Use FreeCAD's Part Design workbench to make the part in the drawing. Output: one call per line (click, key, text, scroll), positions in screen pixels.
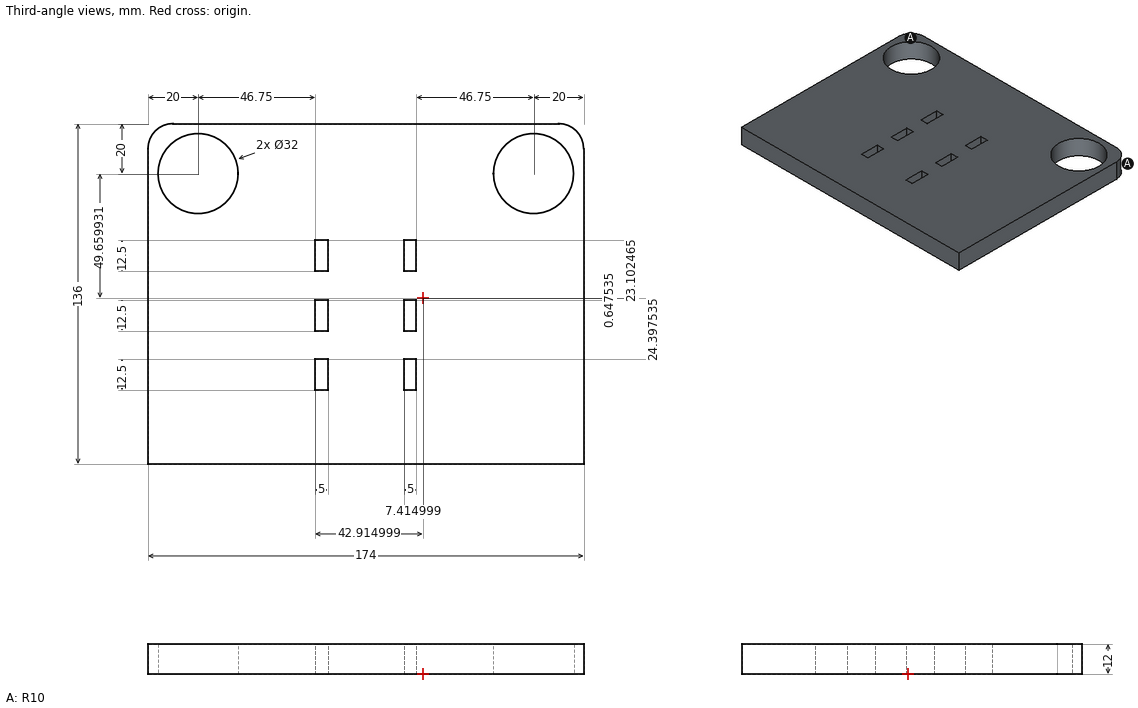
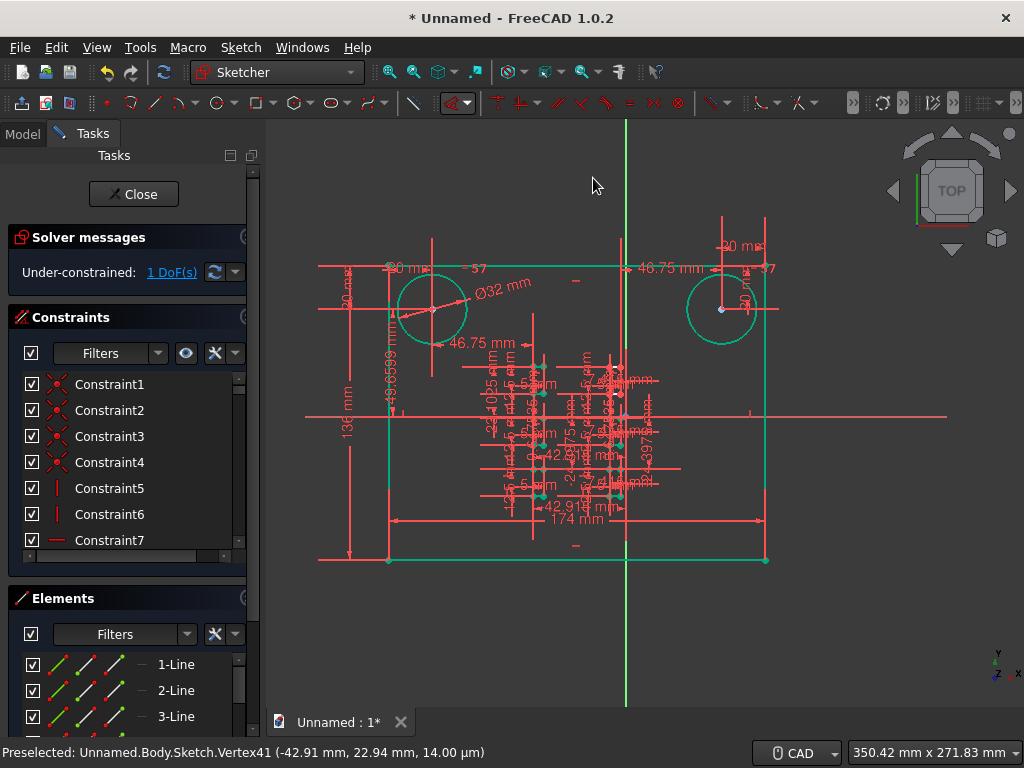
click(610, 367)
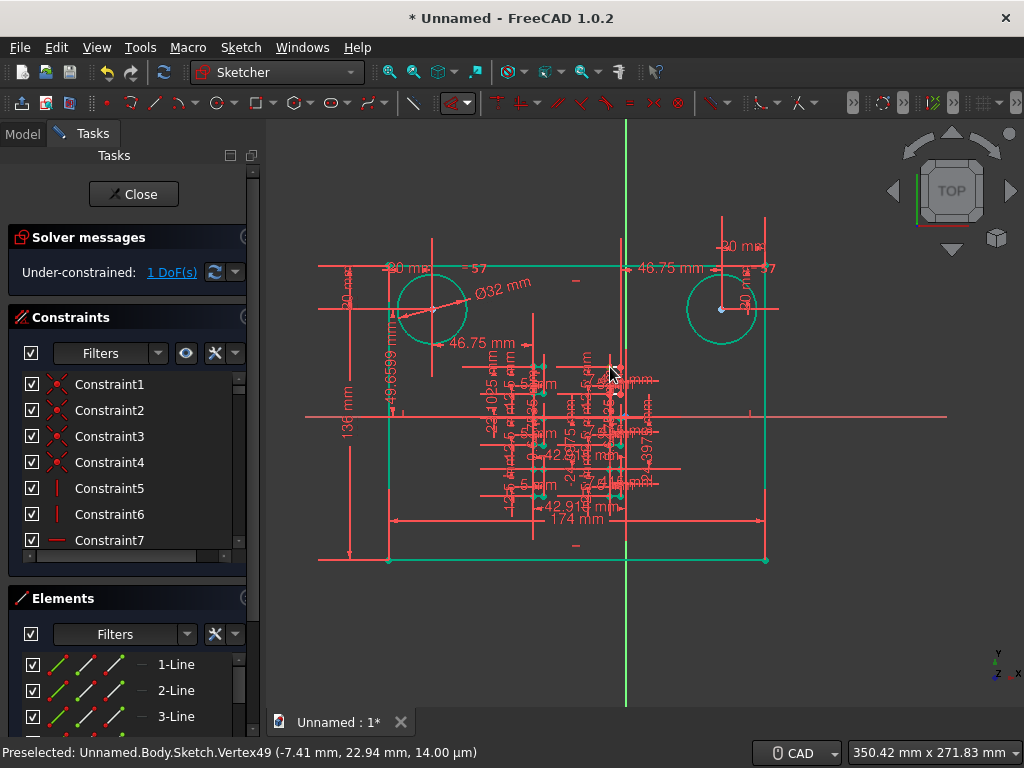
key(i)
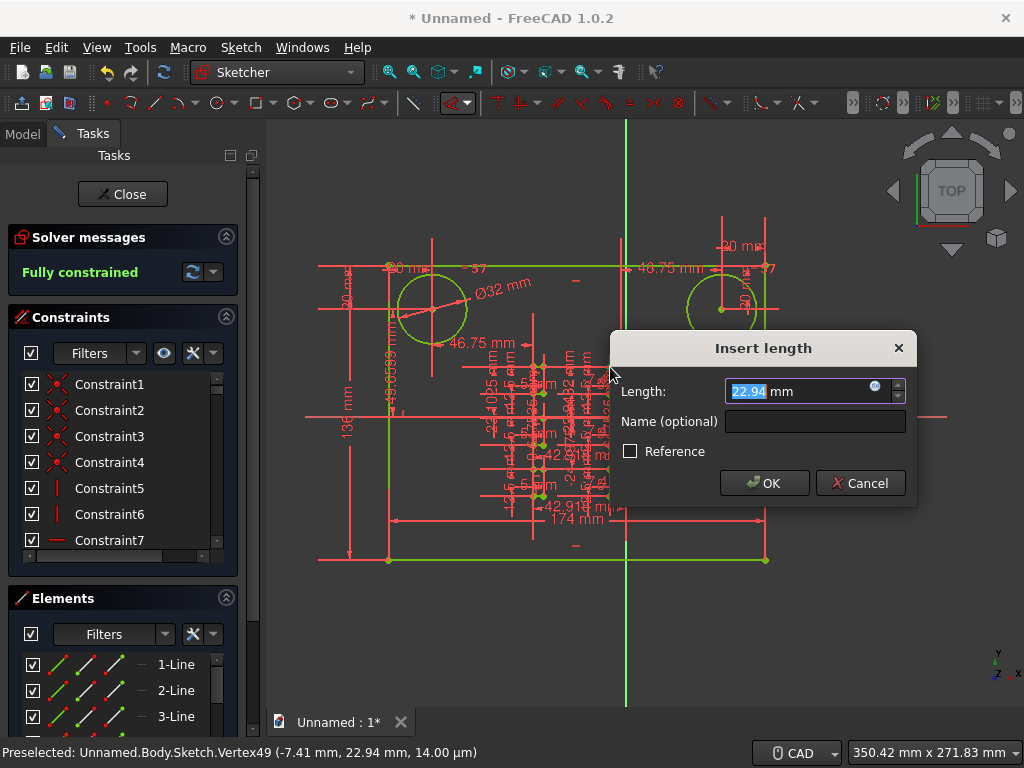
text(23.102465)
key(Return)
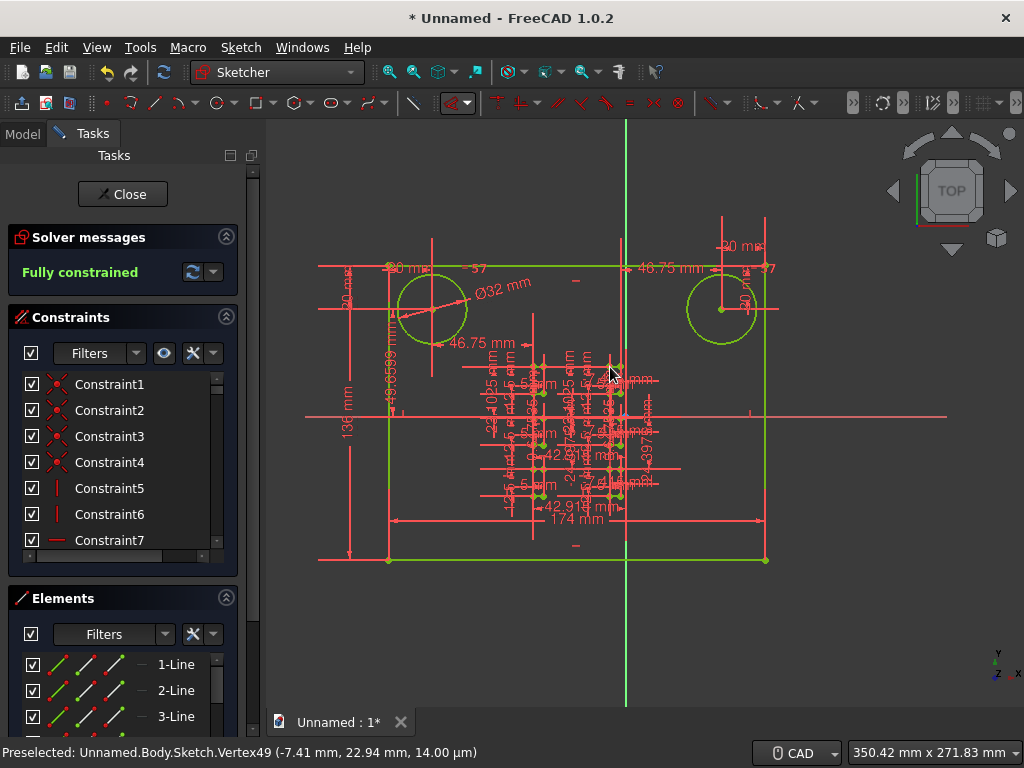
click(123, 194)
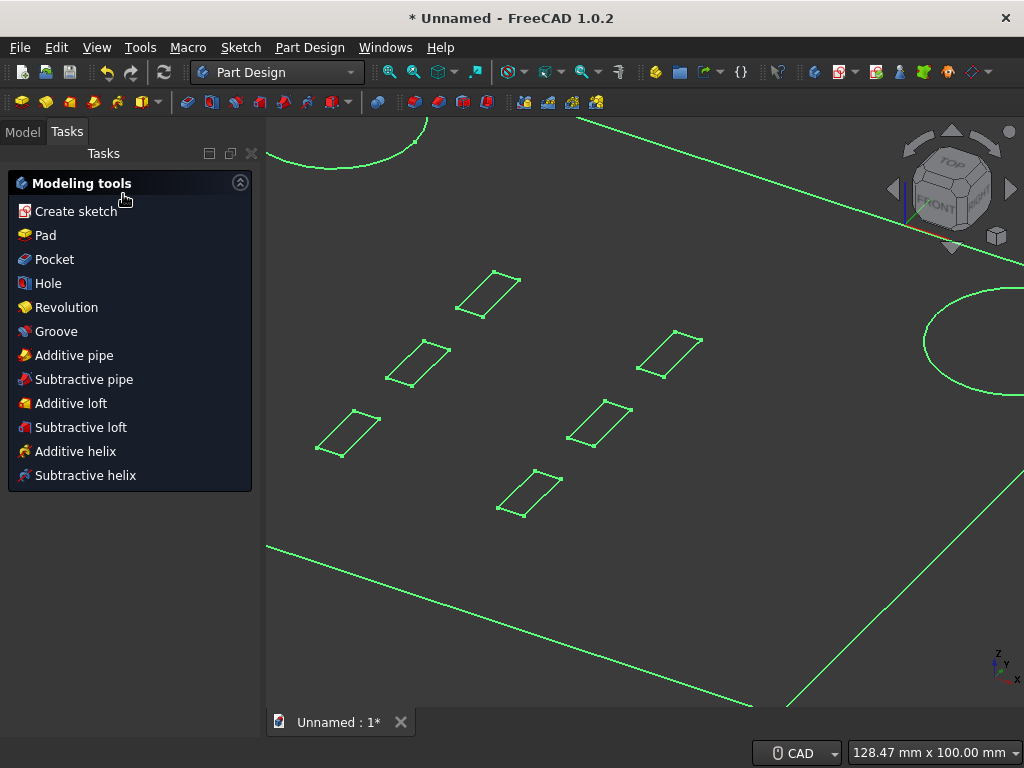
click(22, 102)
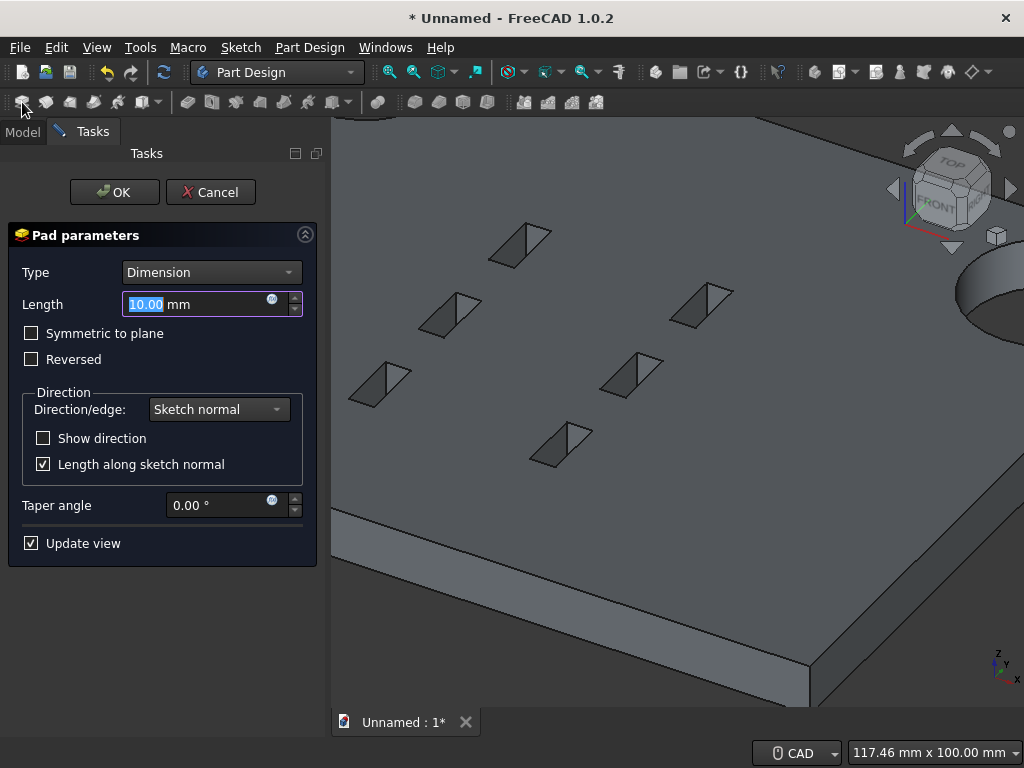
text(12)
key(Tab)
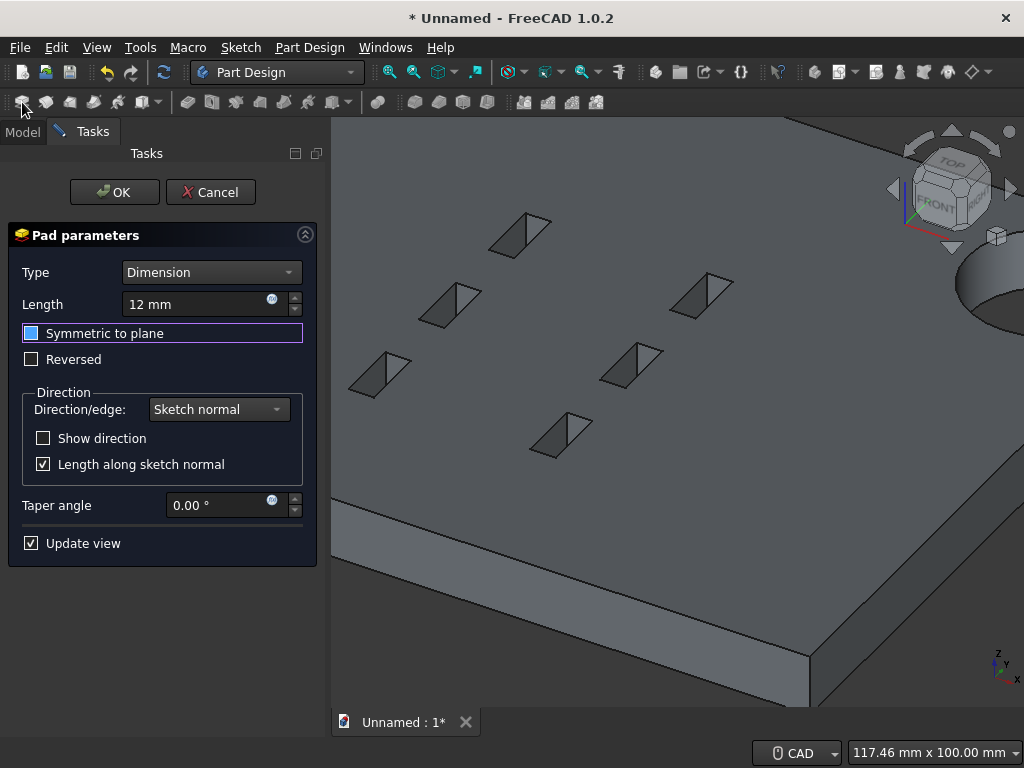
click(115, 192)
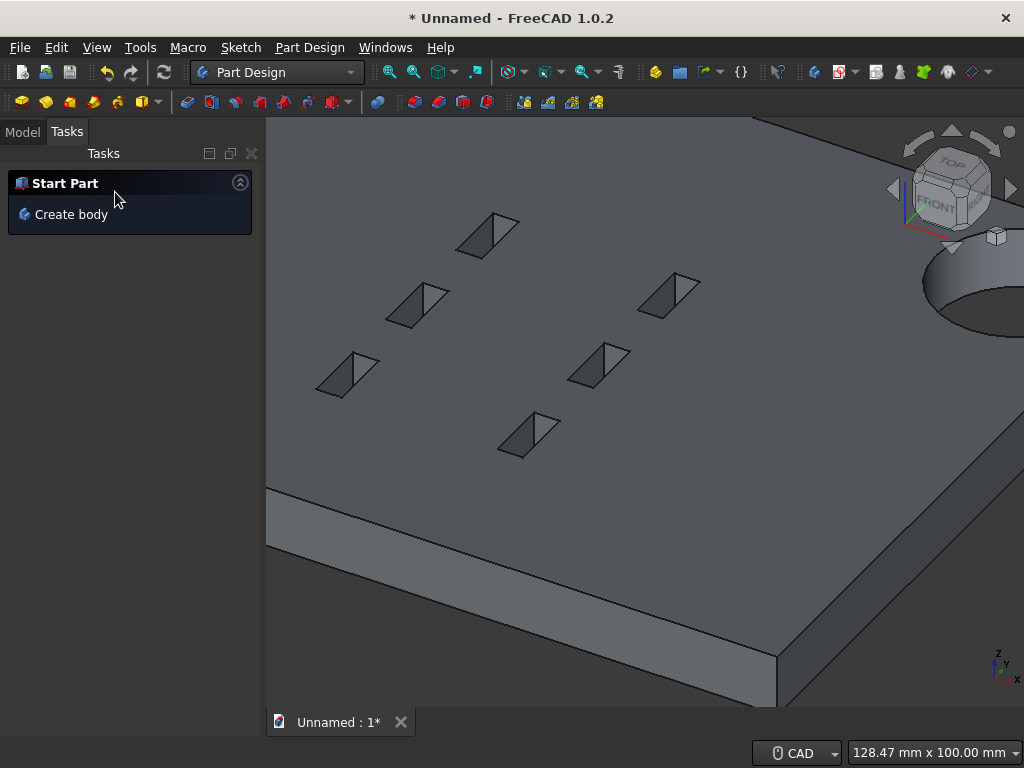
click(390, 72)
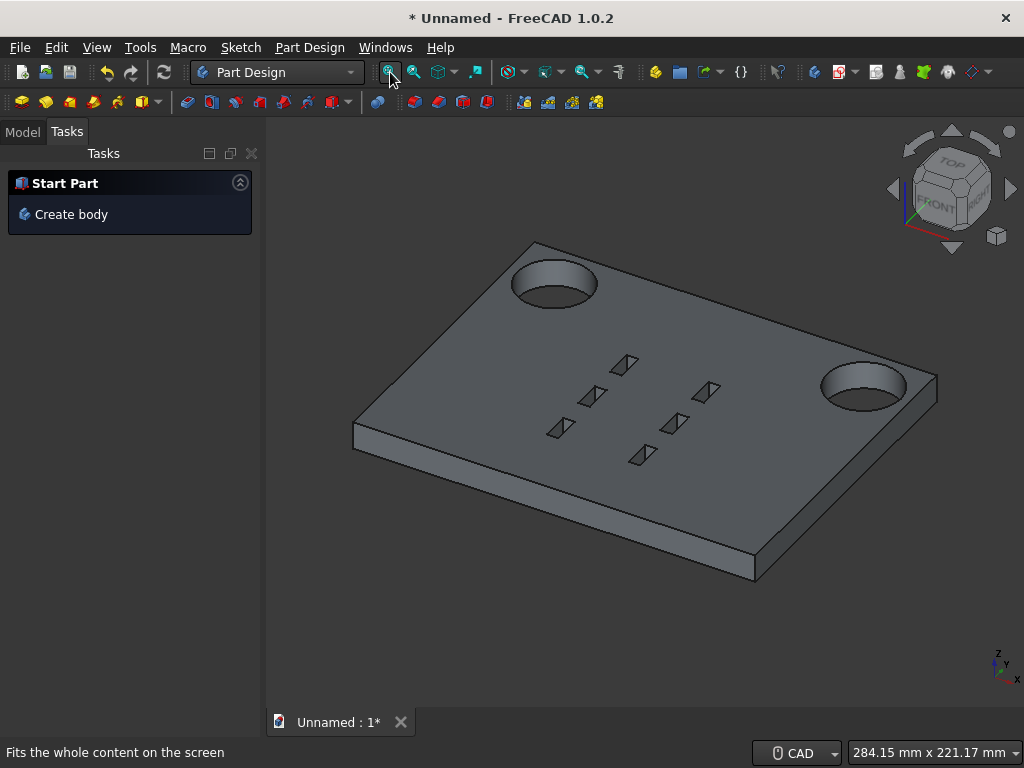
key(0)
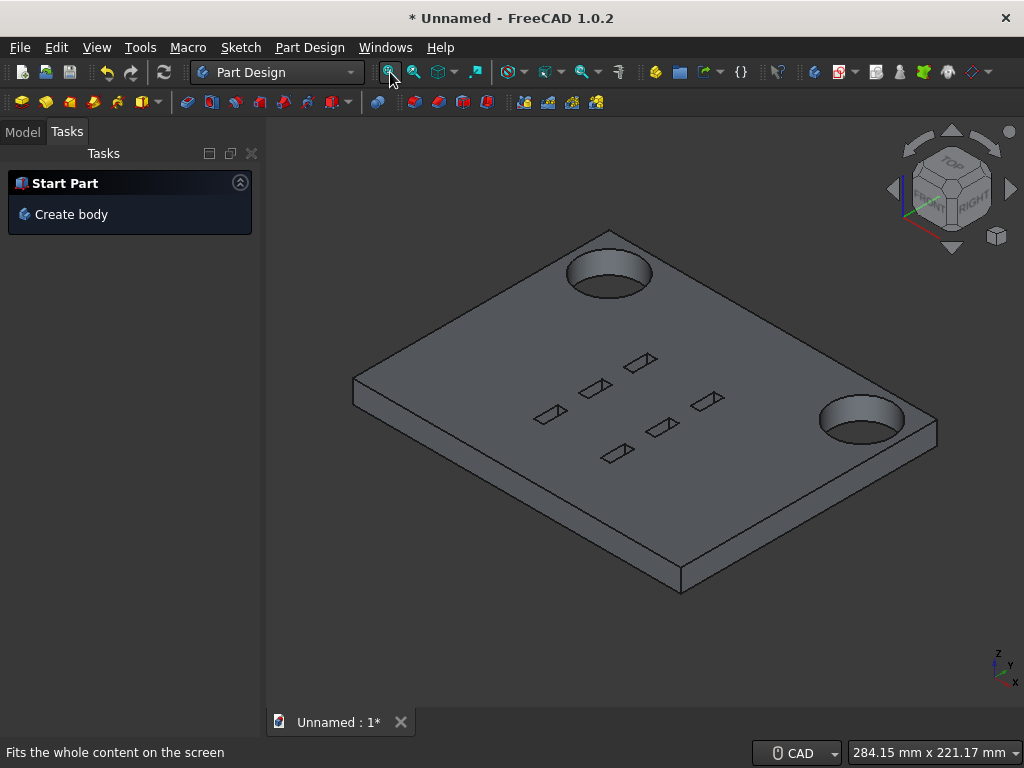
key(2)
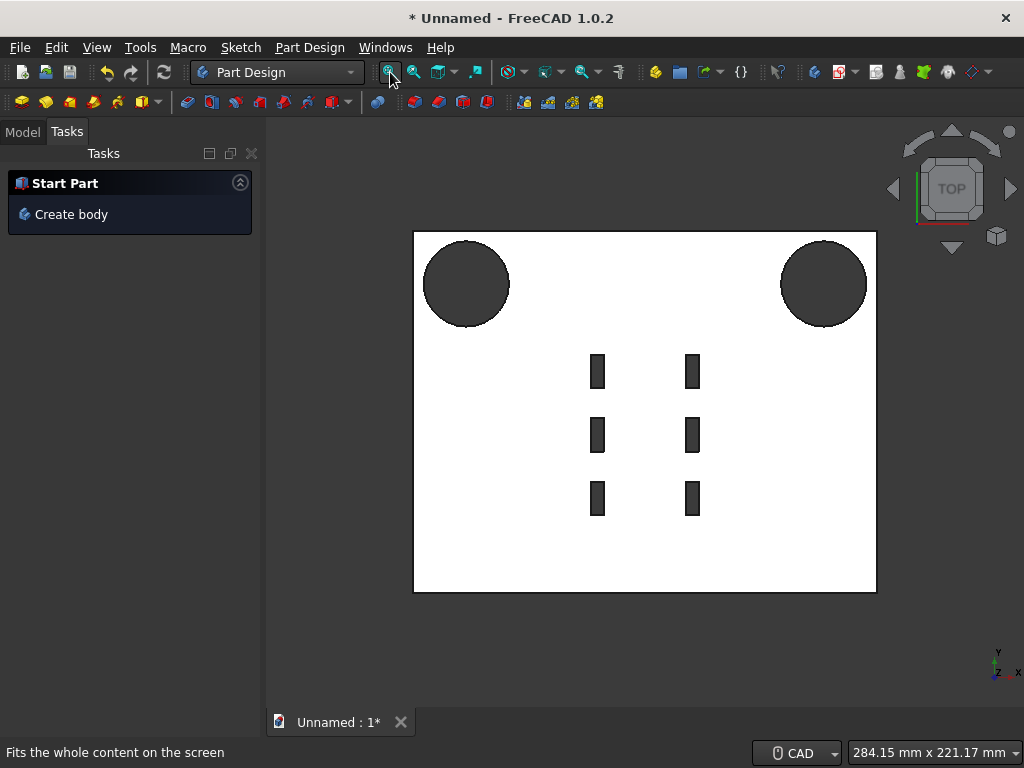
key(1)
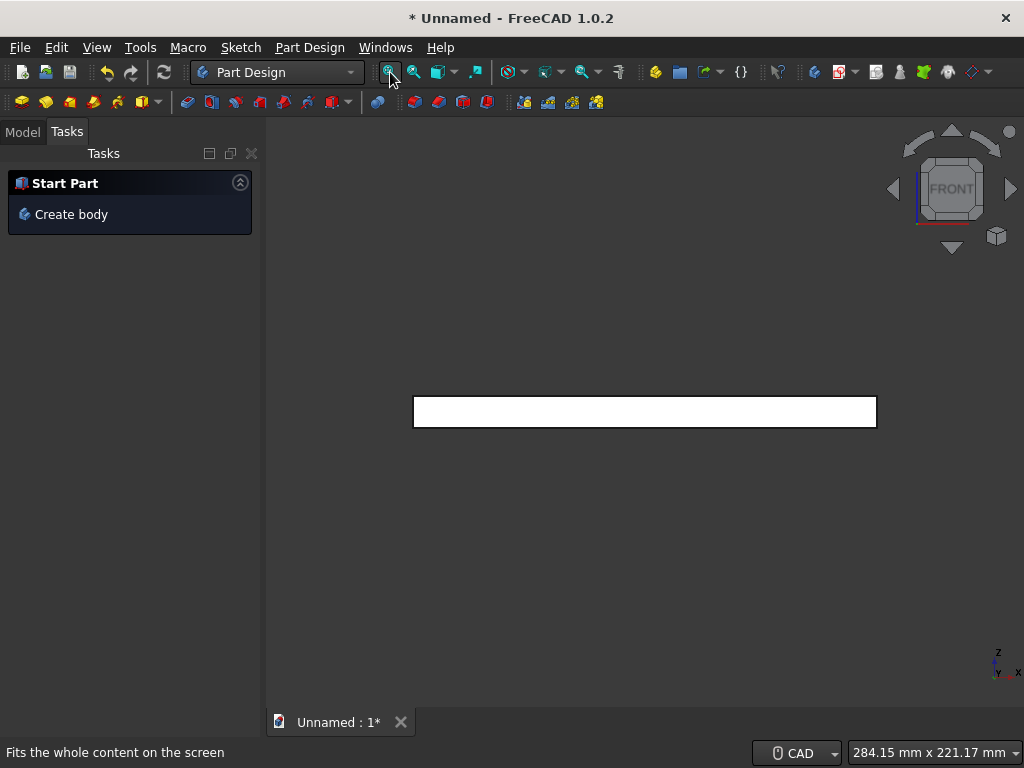
key(3)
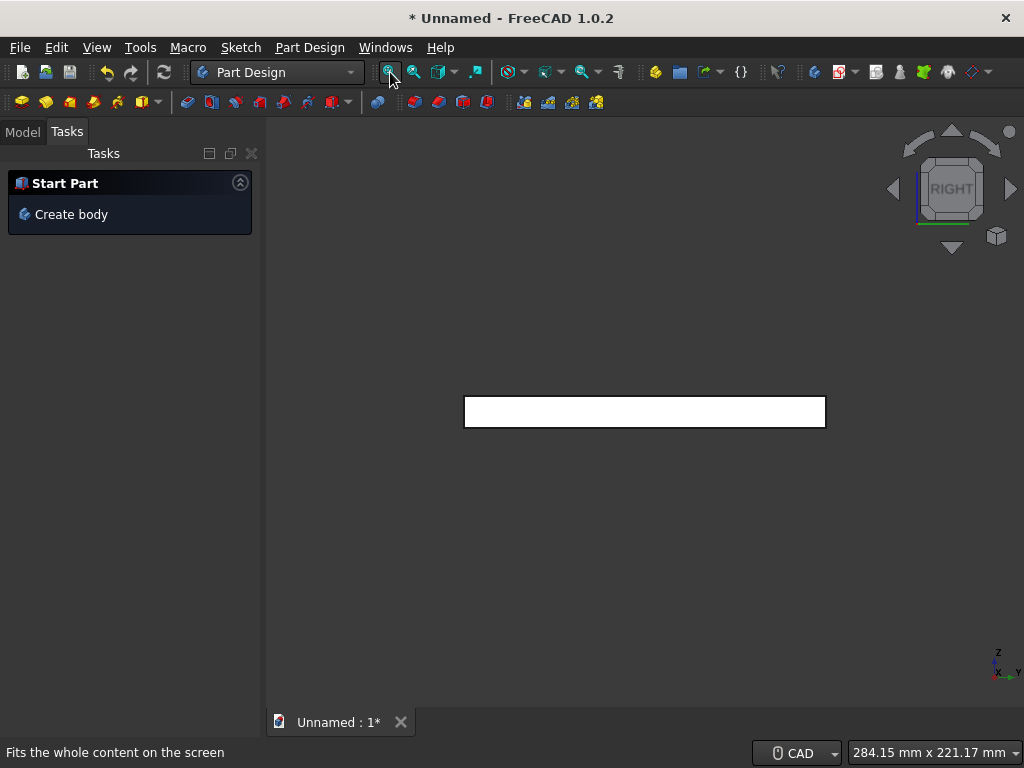
click(826, 411)